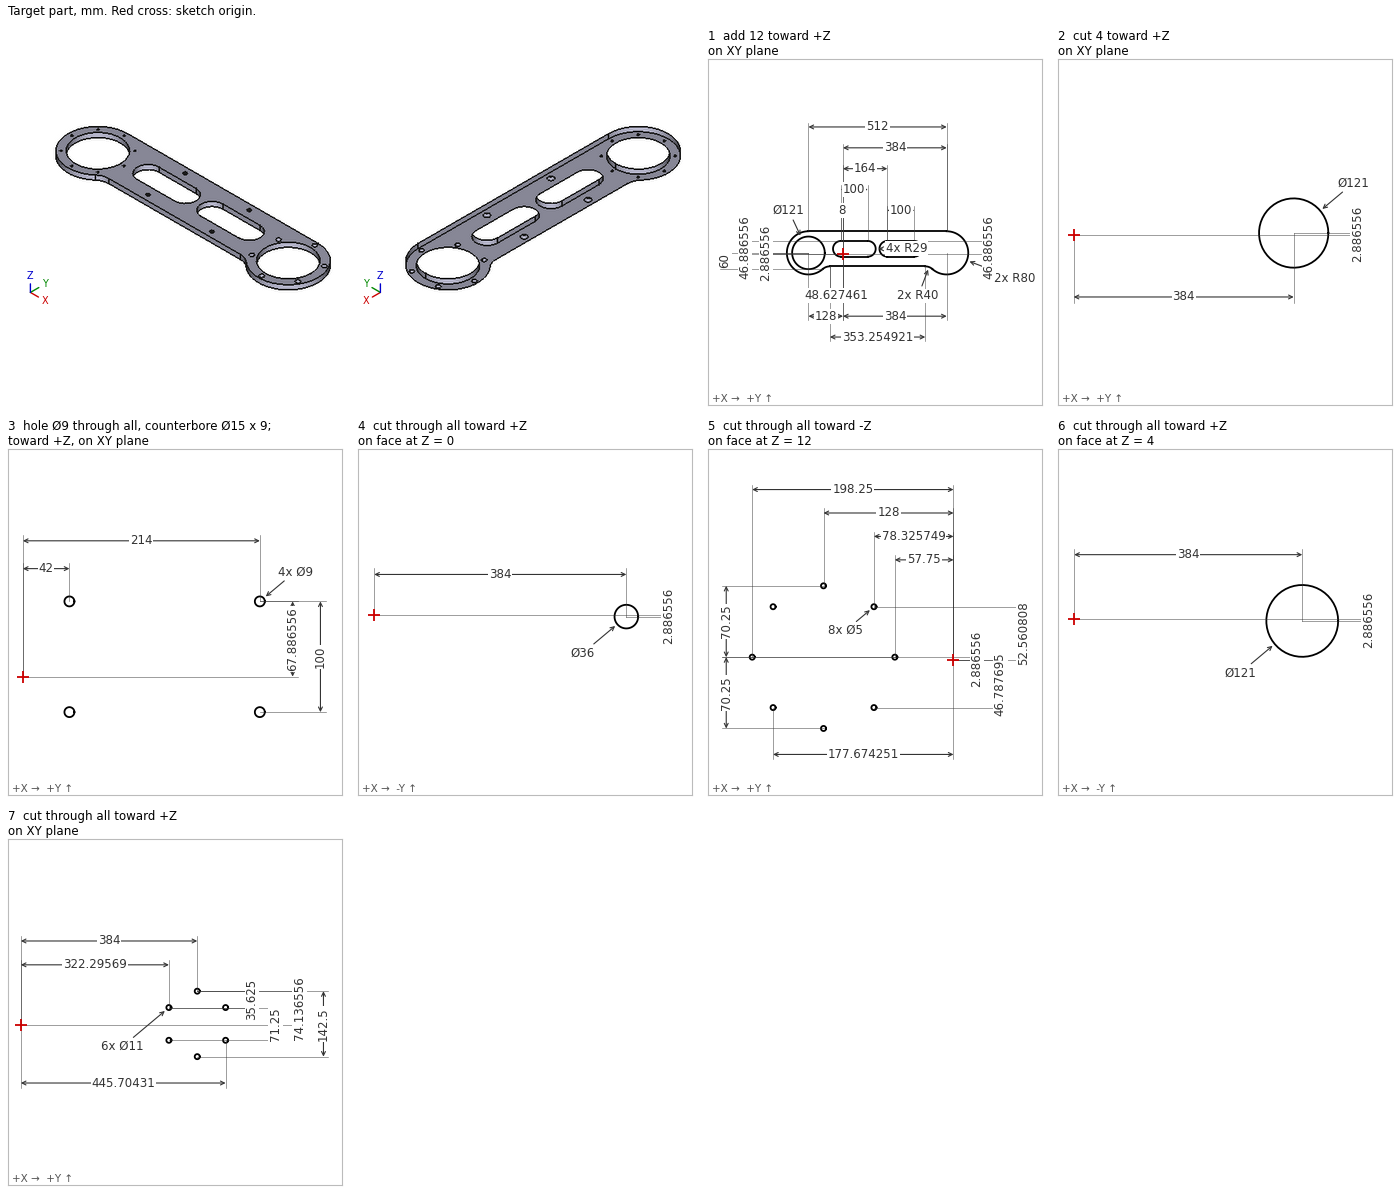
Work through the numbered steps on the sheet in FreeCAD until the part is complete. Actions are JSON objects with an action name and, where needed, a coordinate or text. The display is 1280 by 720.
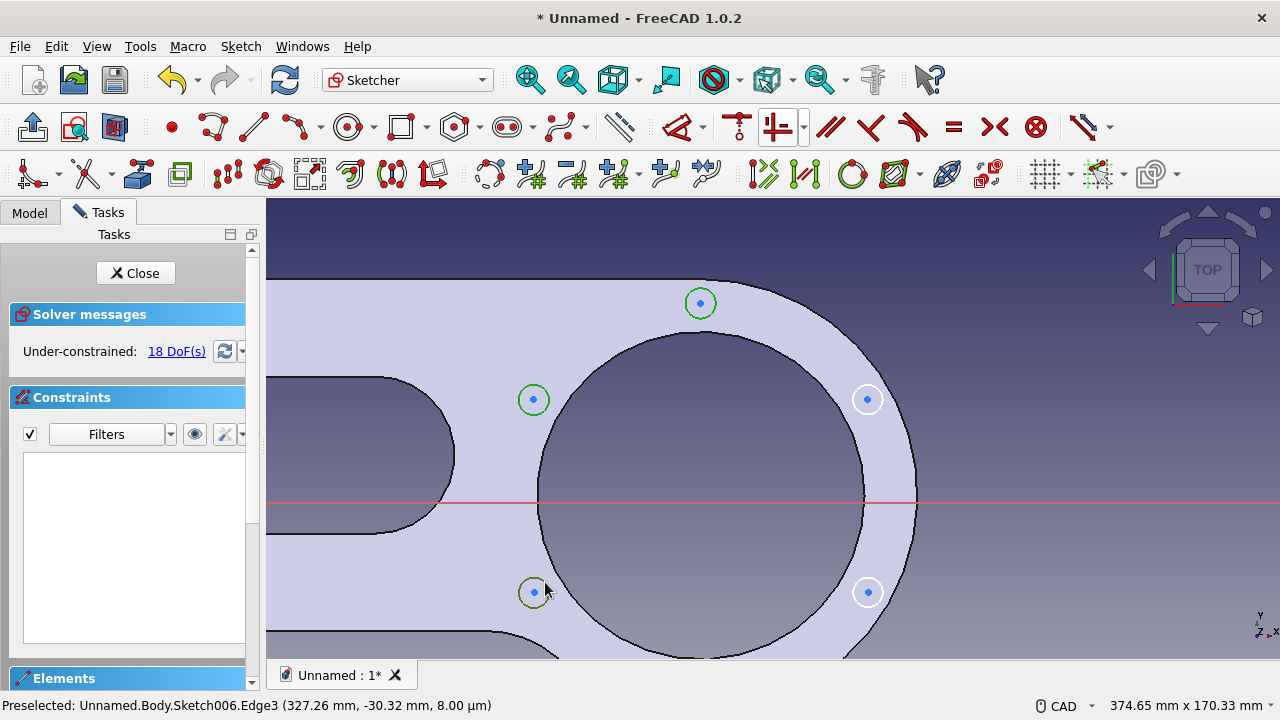
{"action": "scroll", "coordinate": [712, 292], "scroll_direction": "down", "scroll_amount": 2}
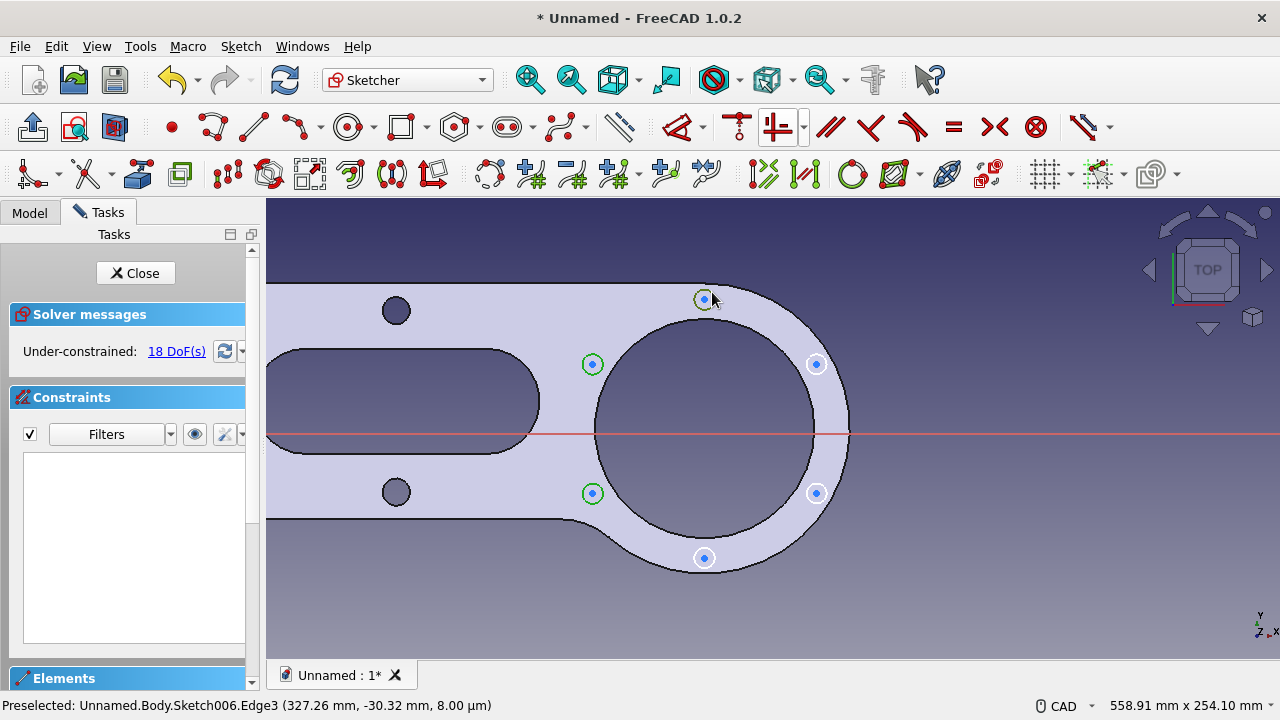
{"action": "scroll", "coordinate": [712, 551], "scroll_direction": "up", "scroll_amount": 2}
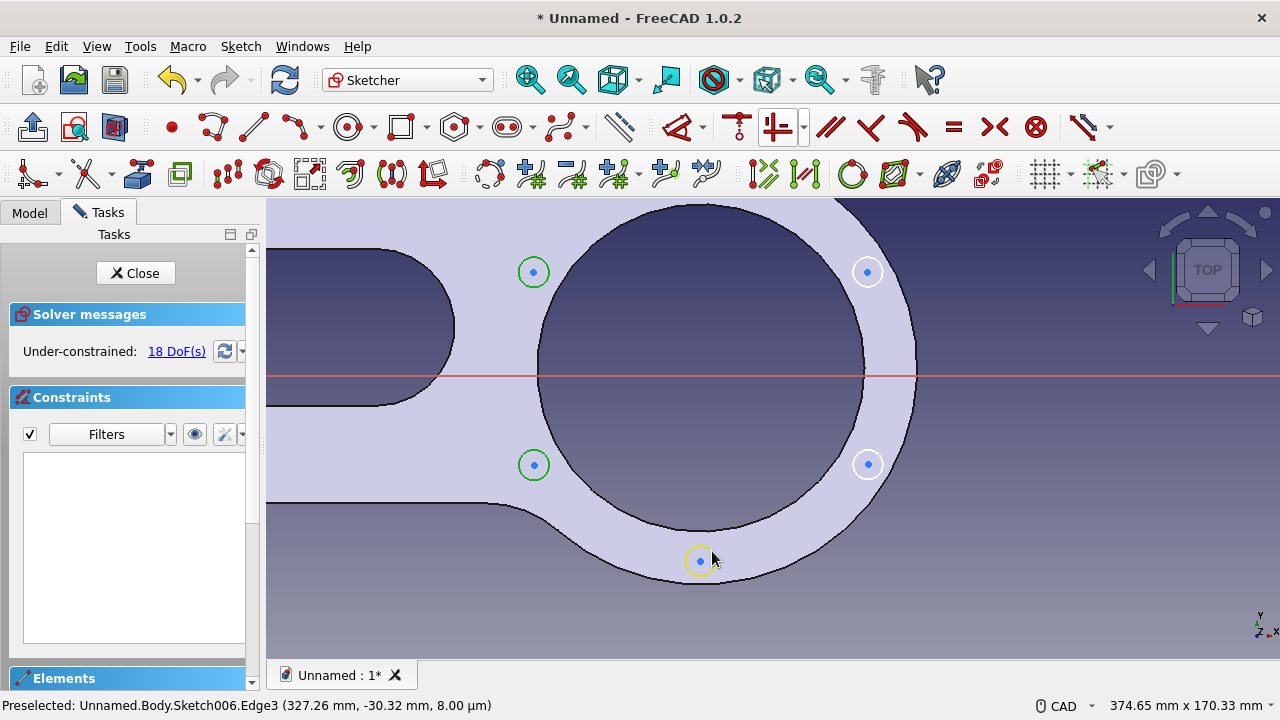
{"action": "left_click", "coordinate": [711, 551]}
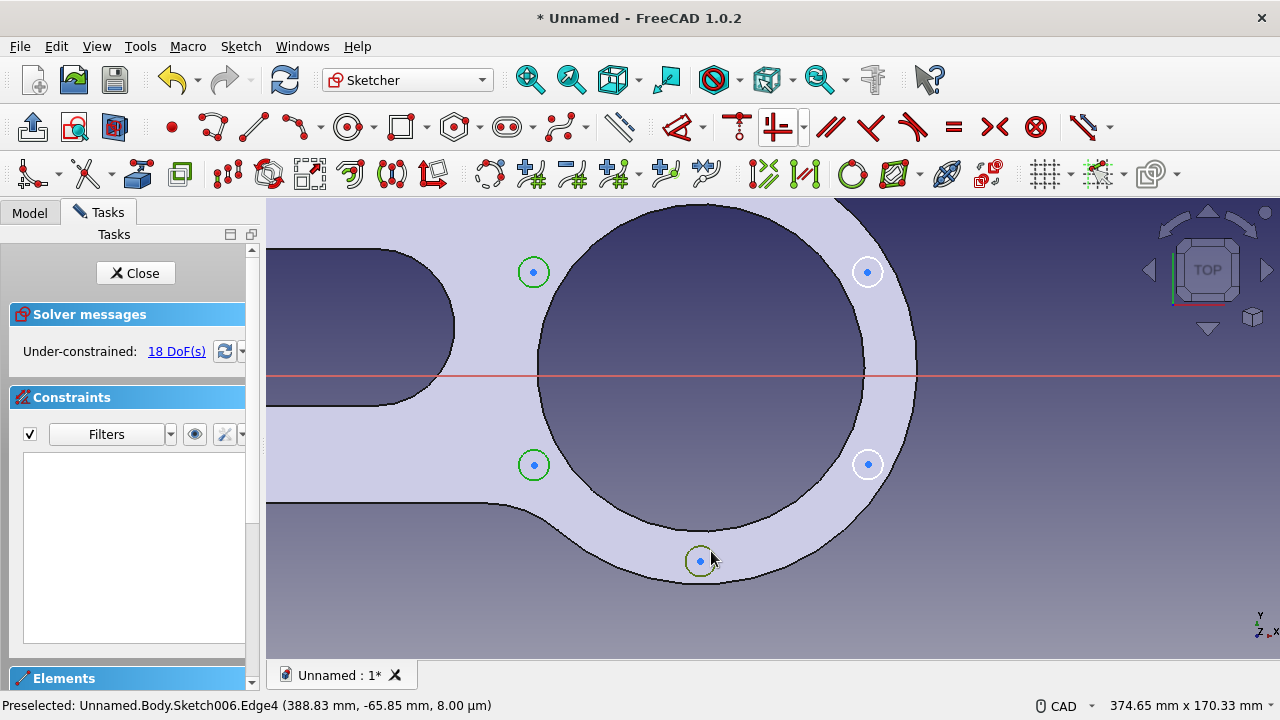
{"action": "left_click", "coordinate": [878, 454]}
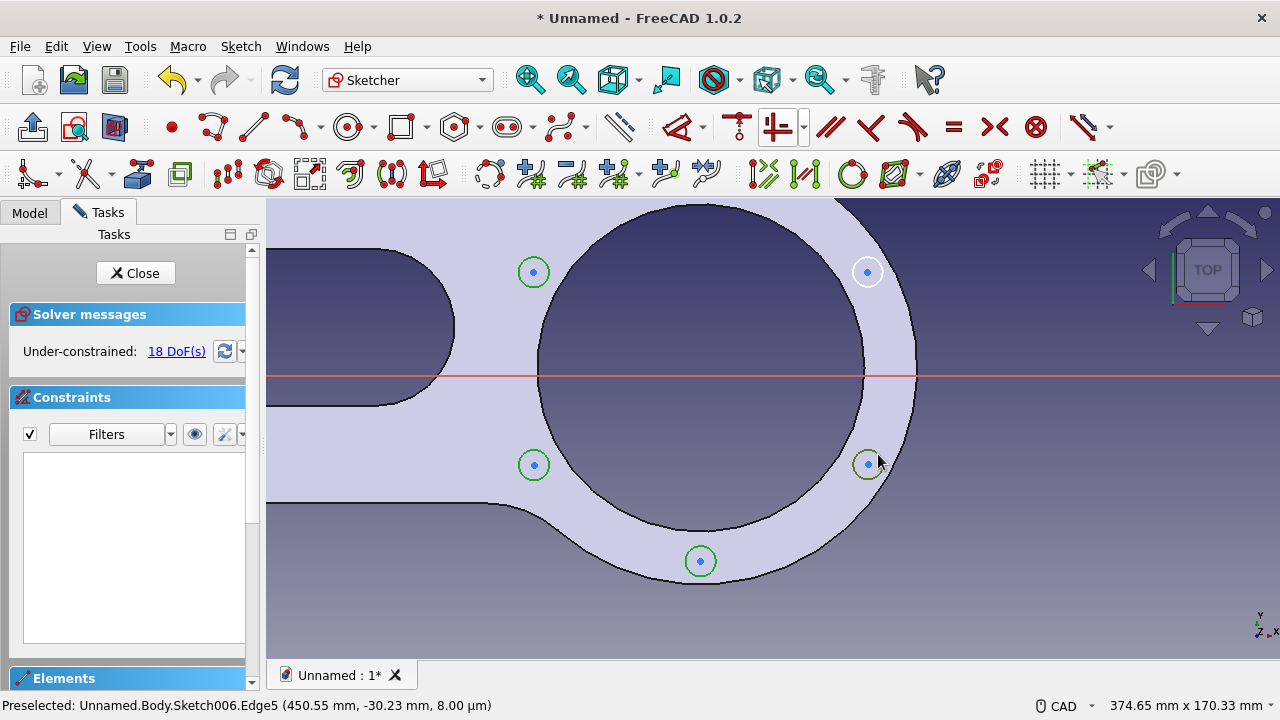
{"action": "left_click", "coordinate": [878, 262]}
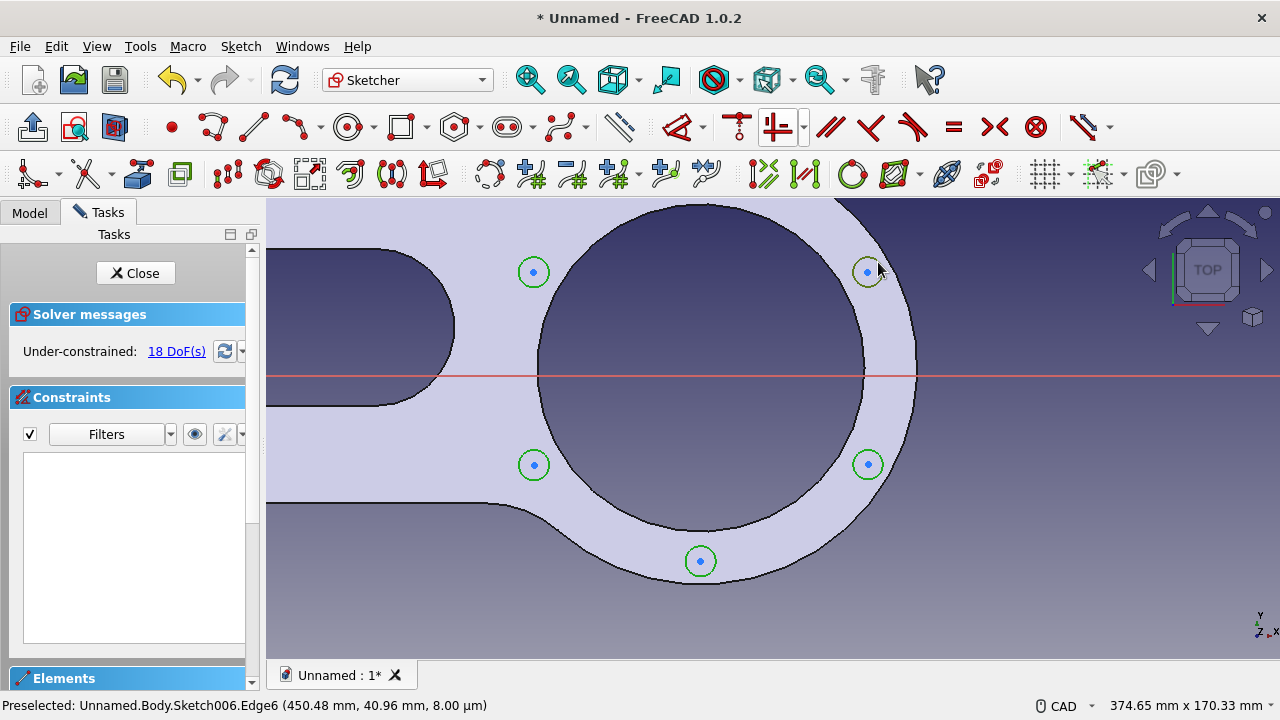
{"action": "left_click", "coordinate": [954, 128]}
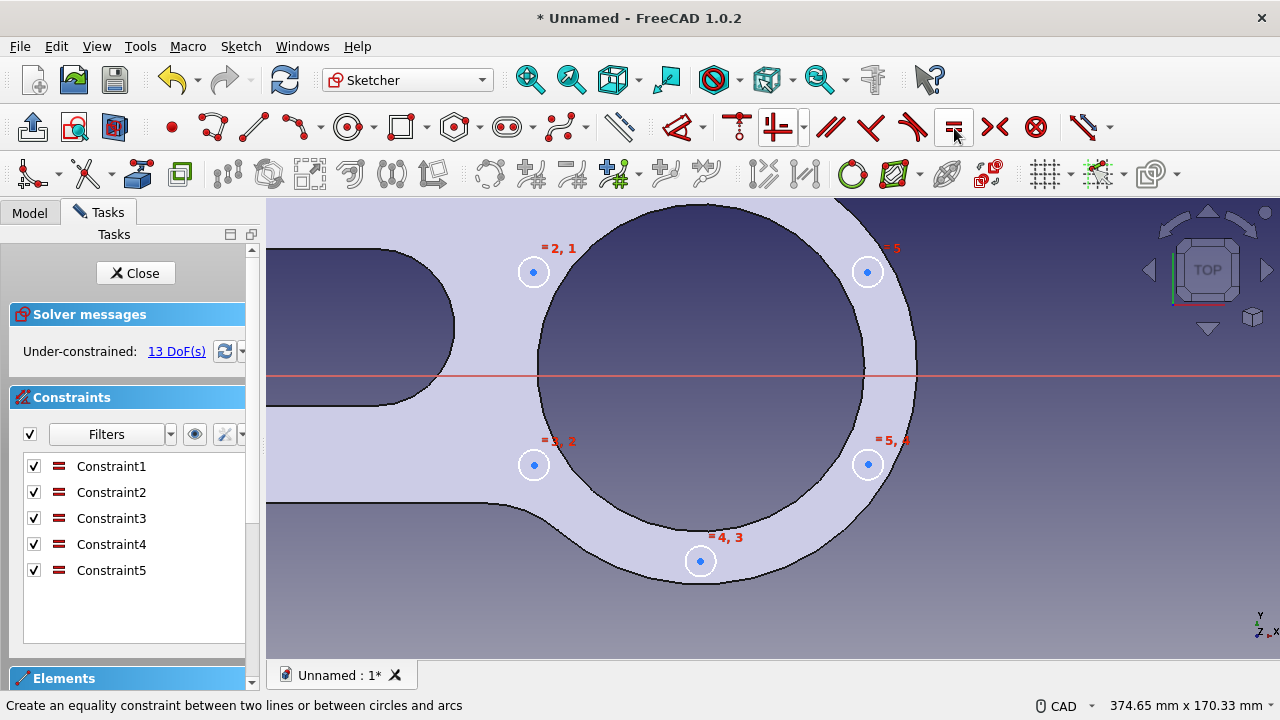
{"action": "left_click", "coordinate": [534, 272]}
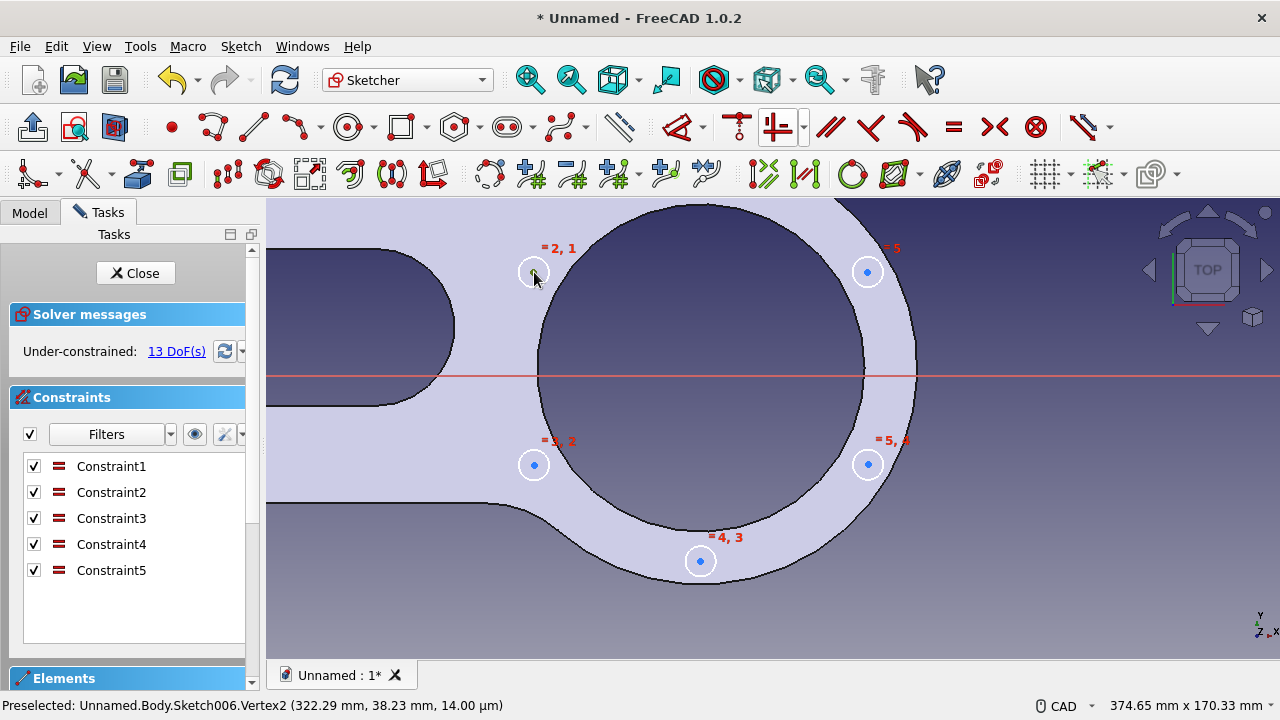
{"action": "left_click", "coordinate": [534, 465]}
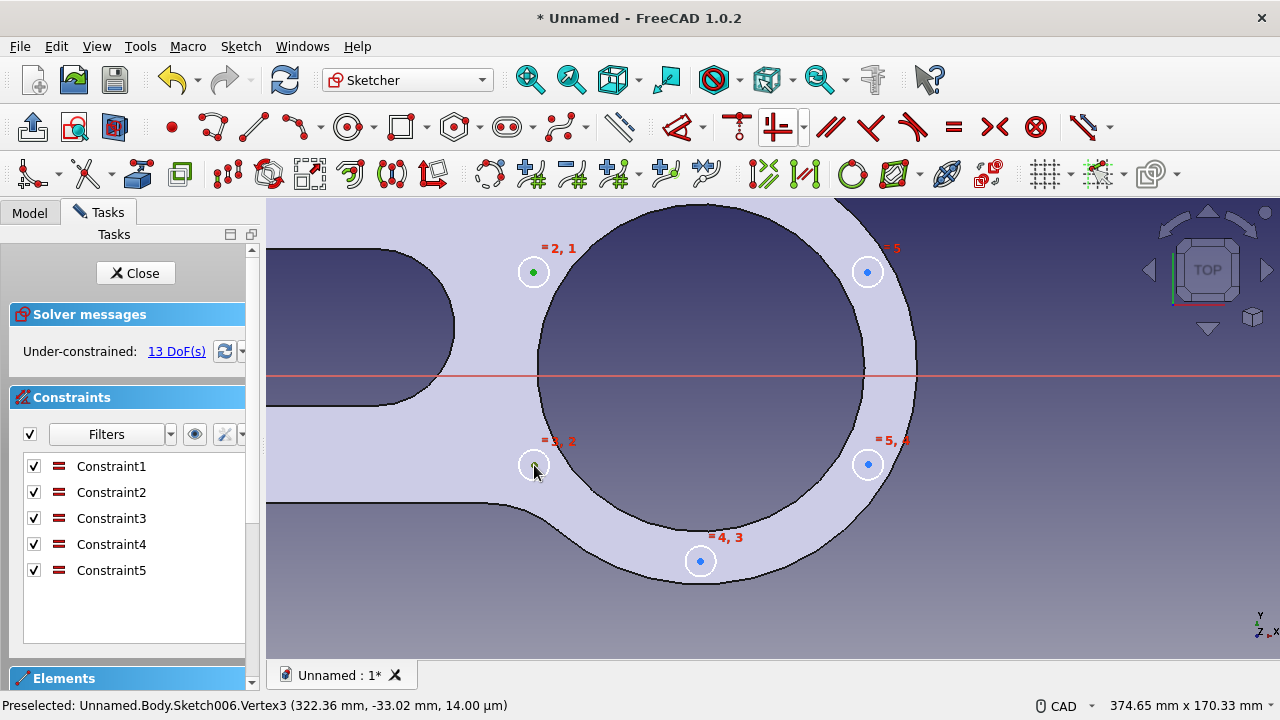
{"action": "key", "text": "v"}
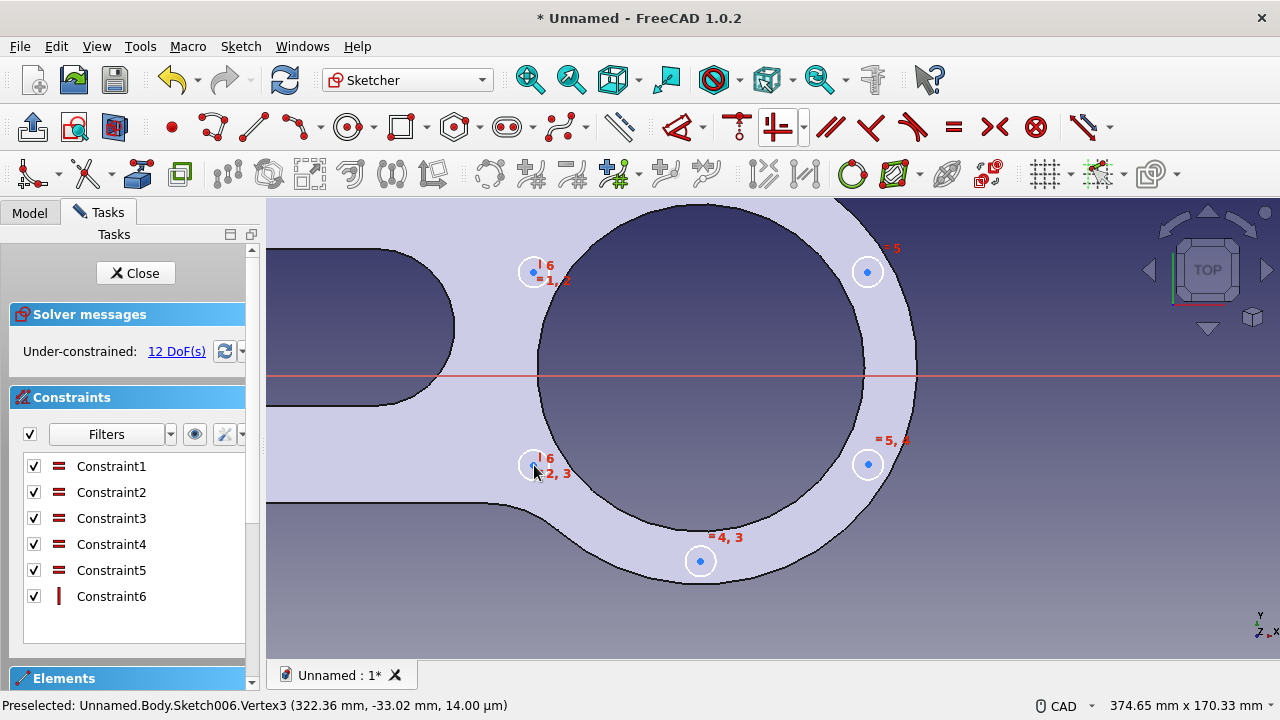
{"action": "scroll", "coordinate": [712, 552], "scroll_direction": "down", "scroll_amount": 2}